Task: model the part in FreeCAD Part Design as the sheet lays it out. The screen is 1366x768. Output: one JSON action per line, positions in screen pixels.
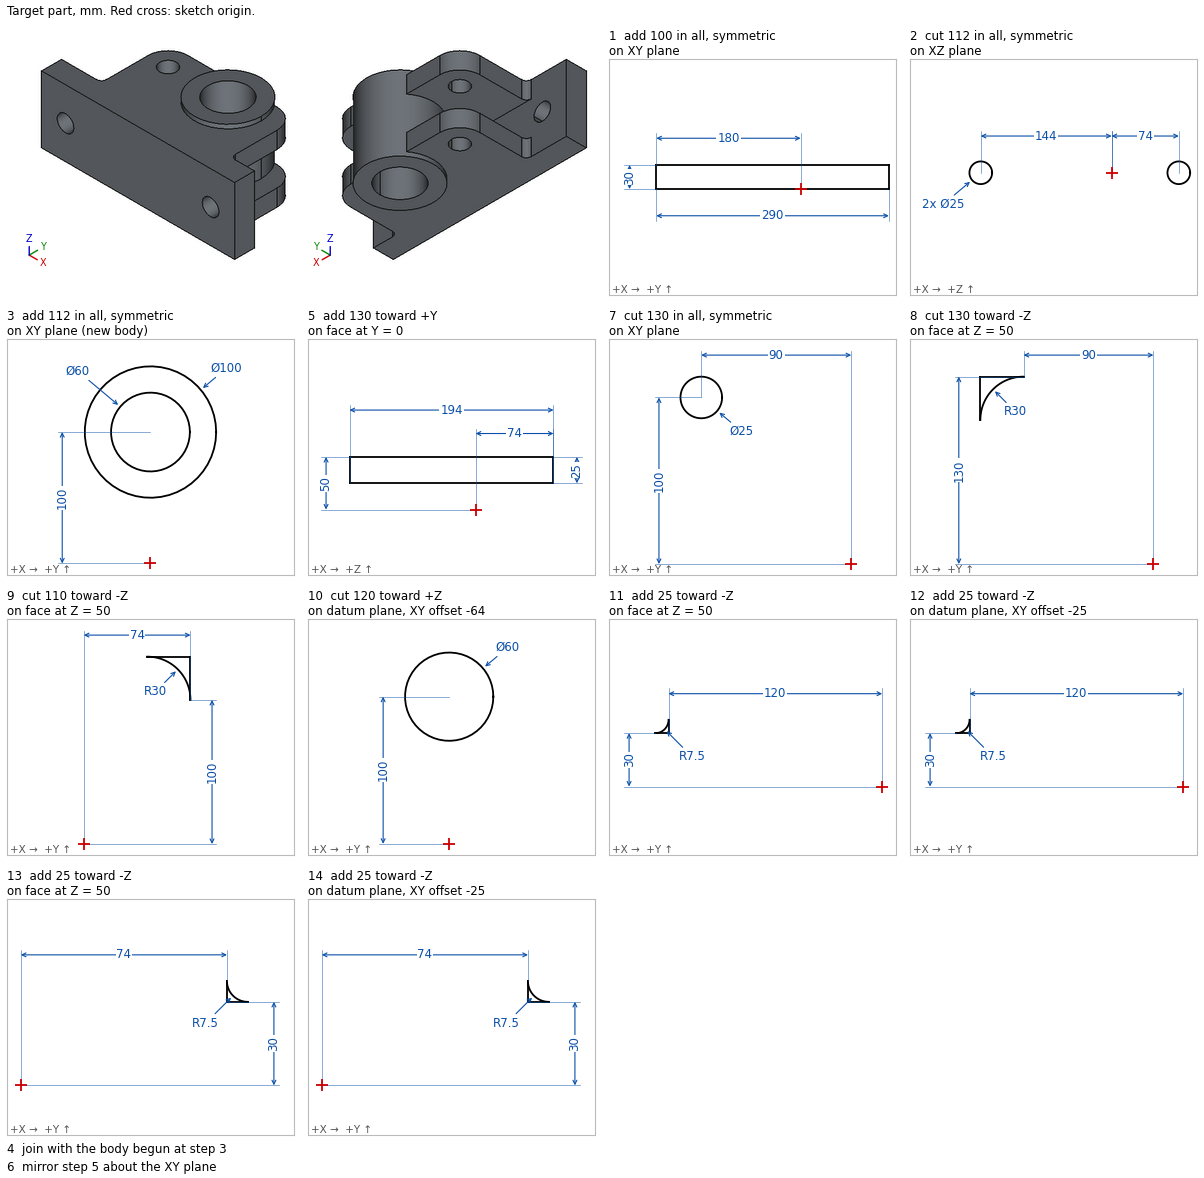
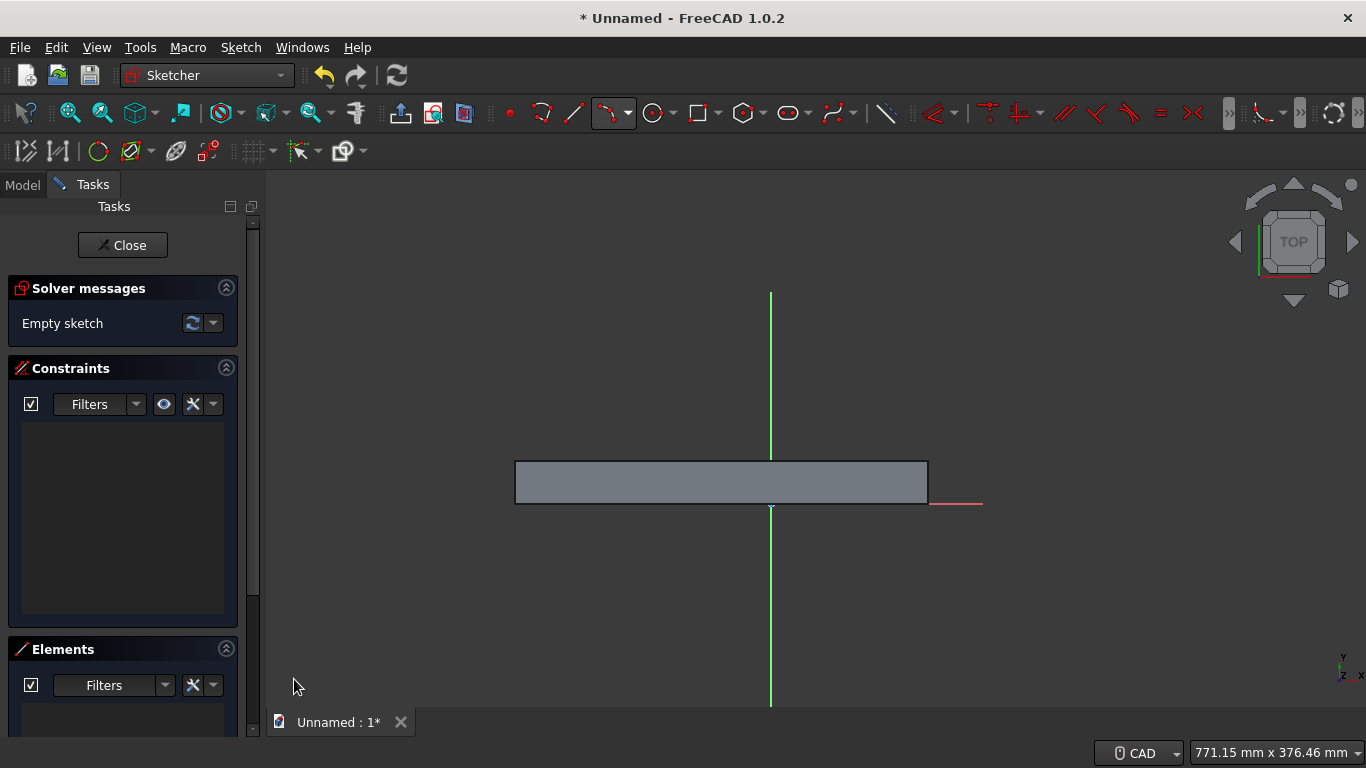
{"action": "scroll", "coordinate": [820, 312], "scroll_direction": "up", "scroll_amount": 2}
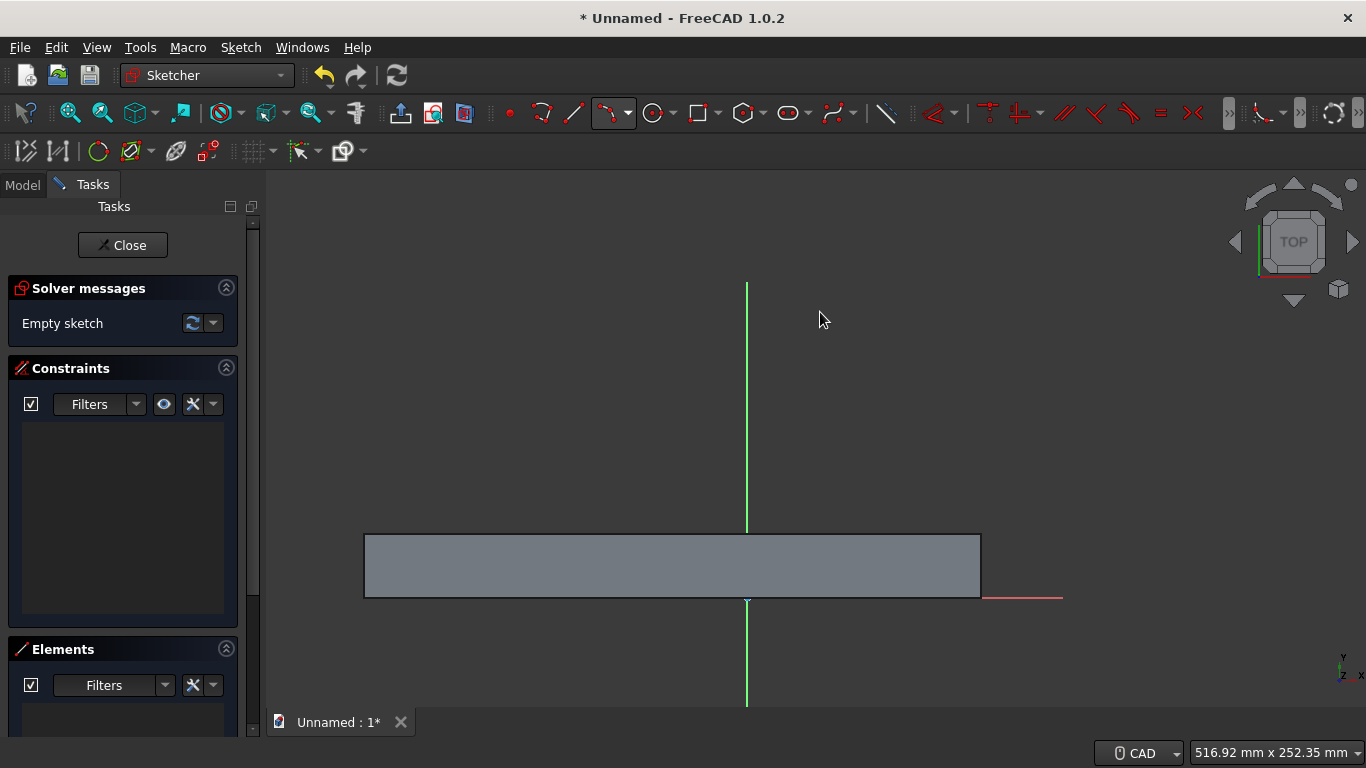
{"action": "left_click", "coordinate": [654, 114]}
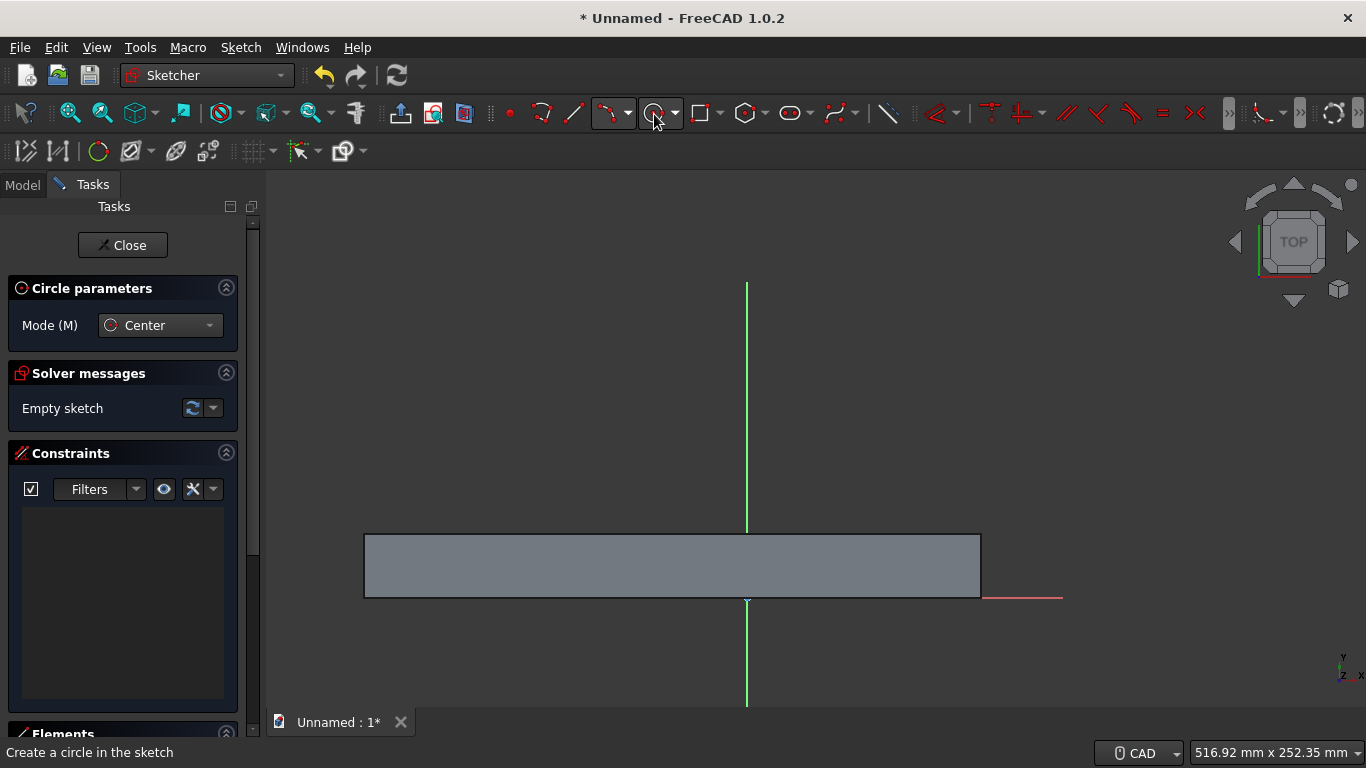
{"action": "left_click", "coordinate": [747, 385]}
{"action": "mouse_move", "coordinate": [822, 310]}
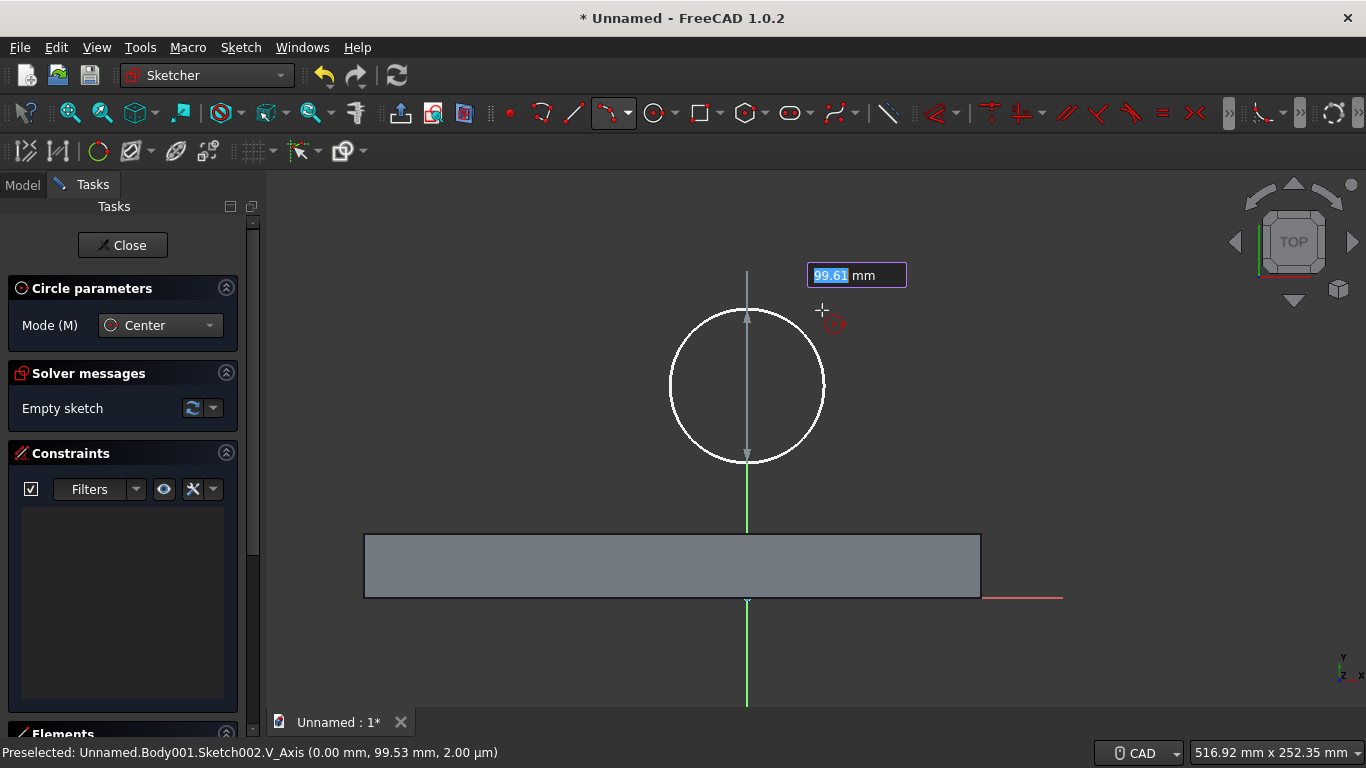
{"action": "type", "text": "100"}
{"action": "key", "text": "Return"}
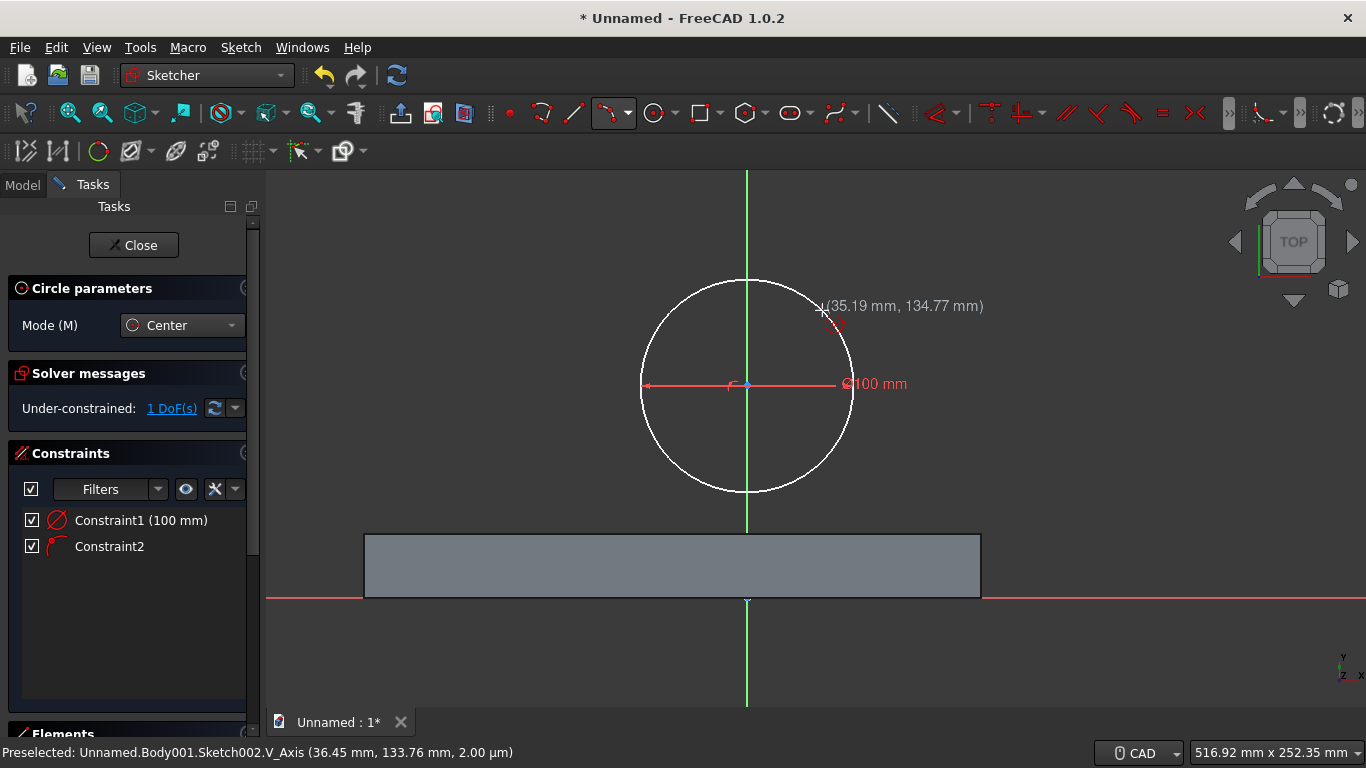
{"action": "left_click", "coordinate": [747, 386]}
{"action": "mouse_move", "coordinate": [792, 340]}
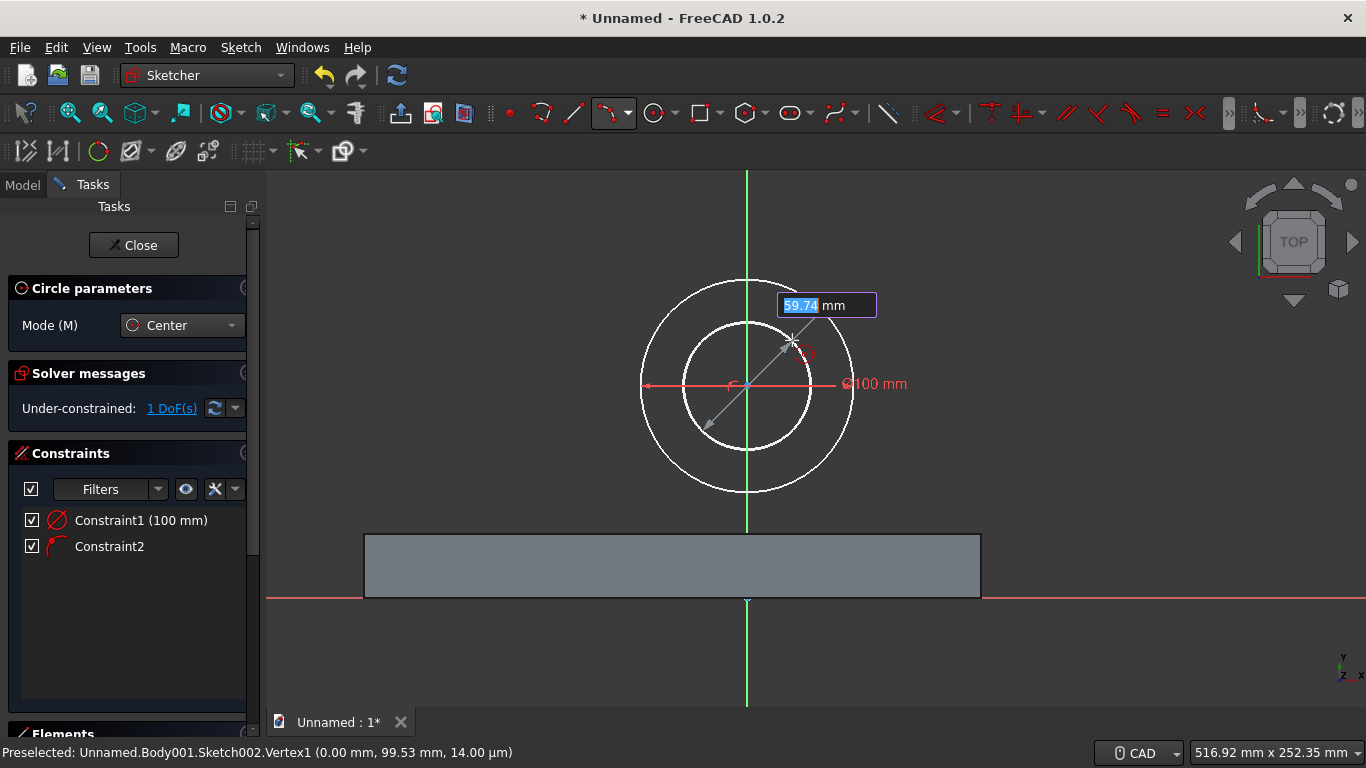
{"action": "type", "text": "60"}
{"action": "key", "text": "Return"}
{"action": "key", "text": "Escape"}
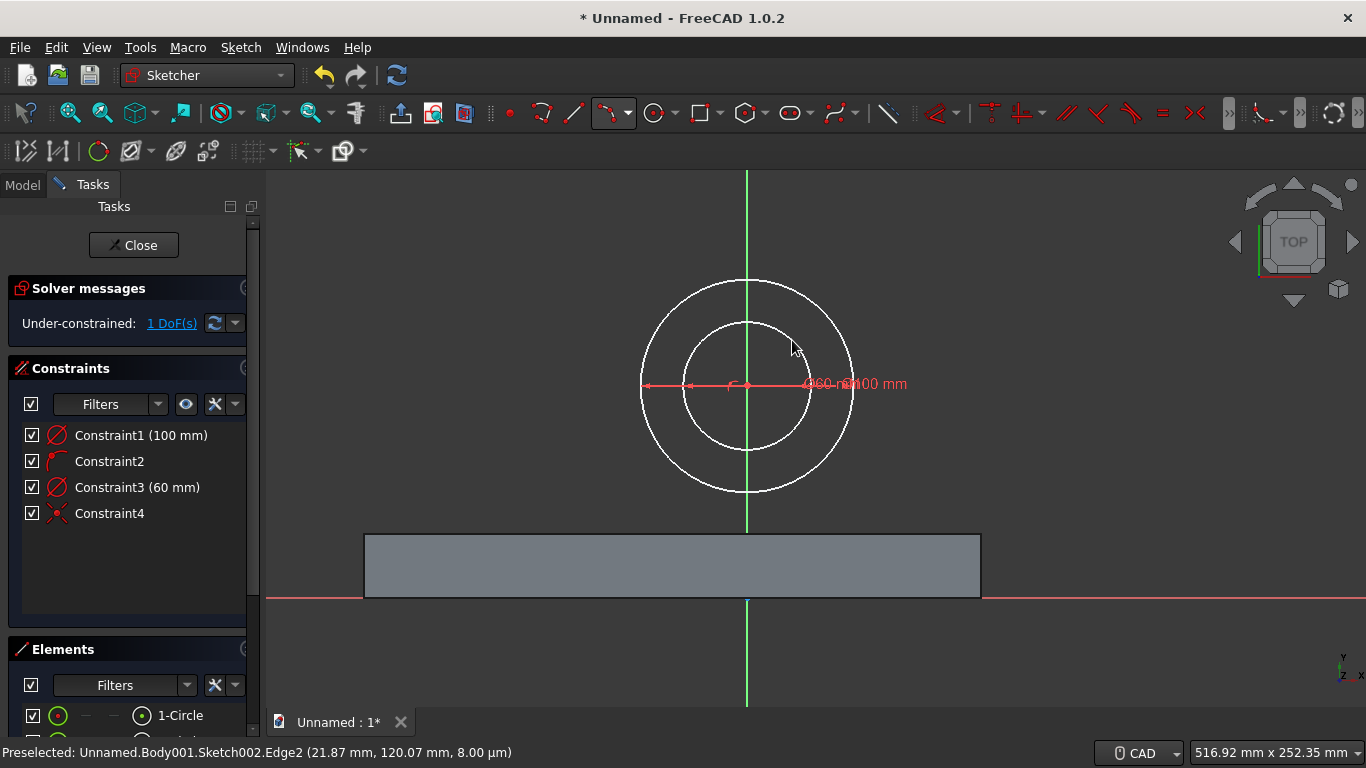
{"action": "left_click", "coordinate": [936, 114]}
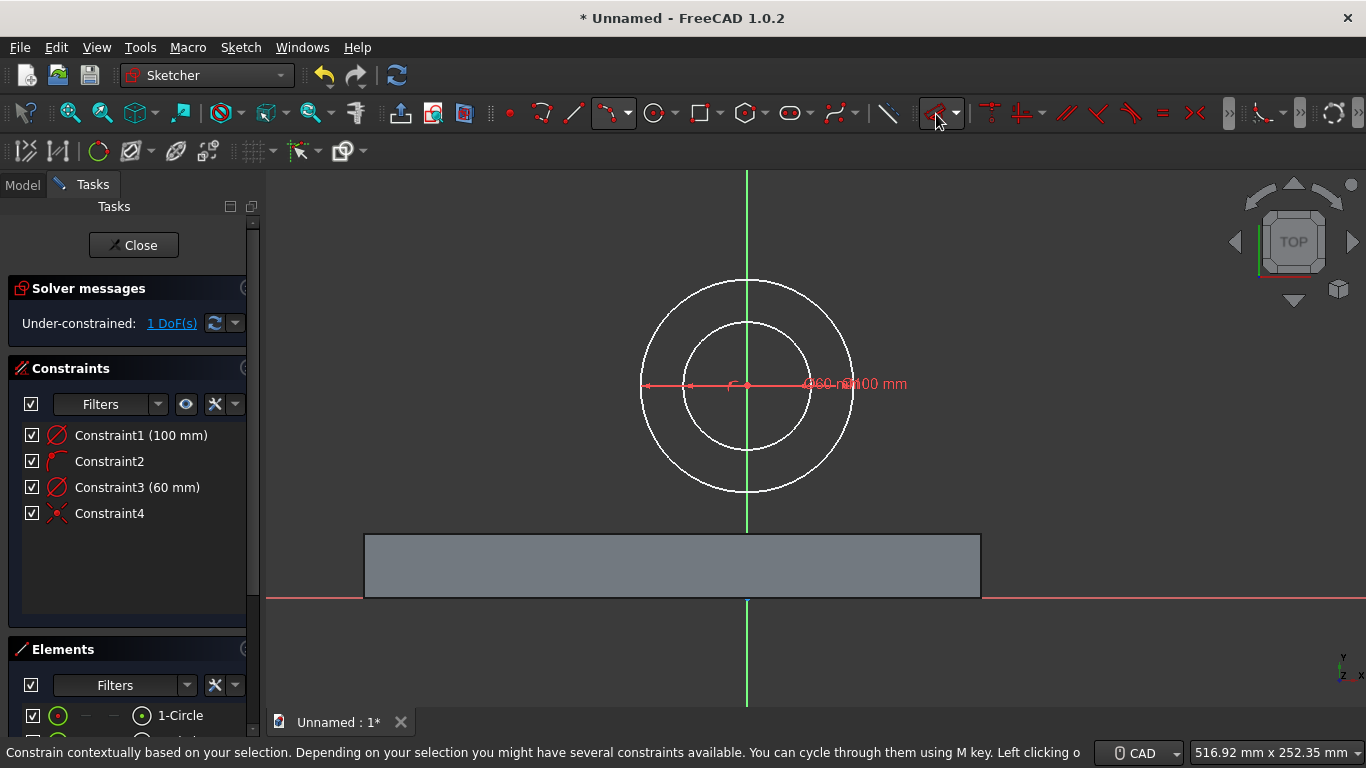
{"action": "left_click", "coordinate": [747, 386]}
{"action": "left_click", "coordinate": [781, 541]}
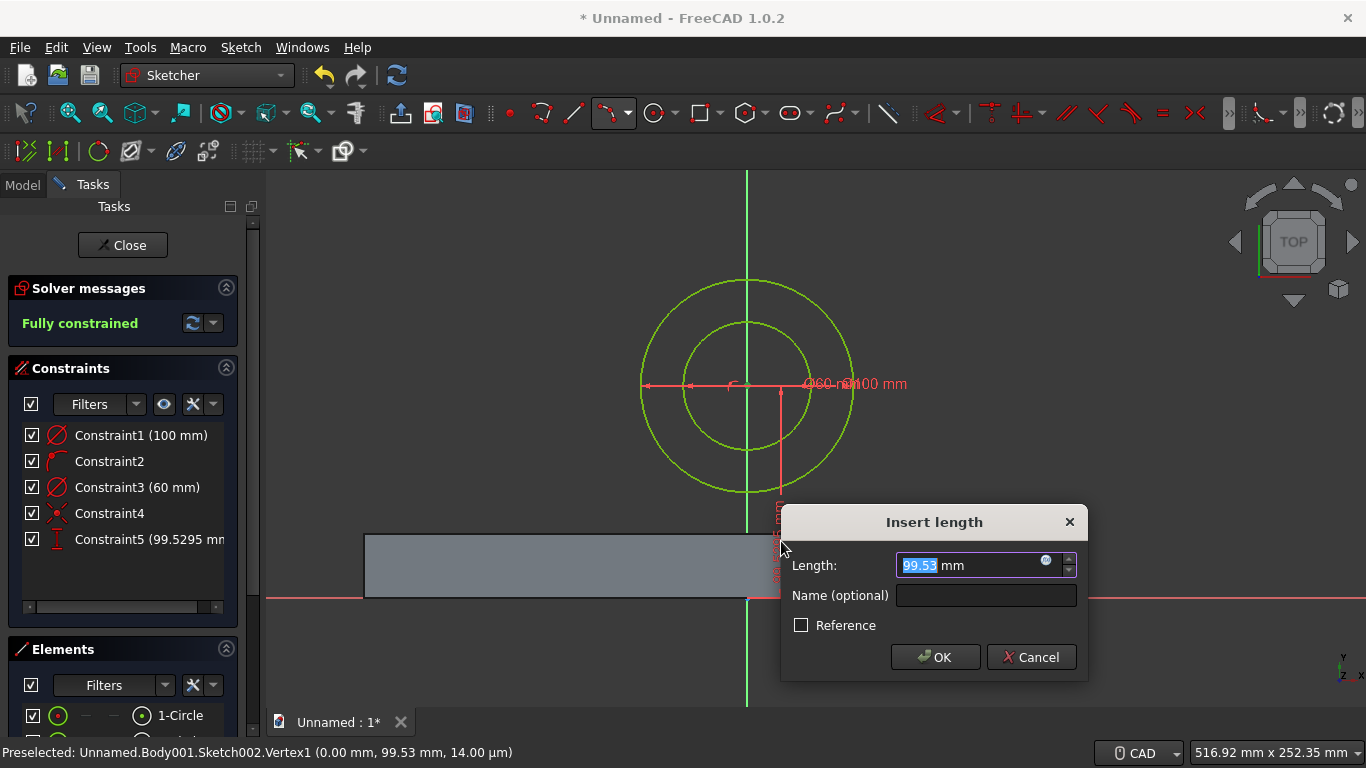
{"action": "type", "text": "100"}
{"action": "key", "text": "Return"}
{"action": "key", "text": "Escape"}